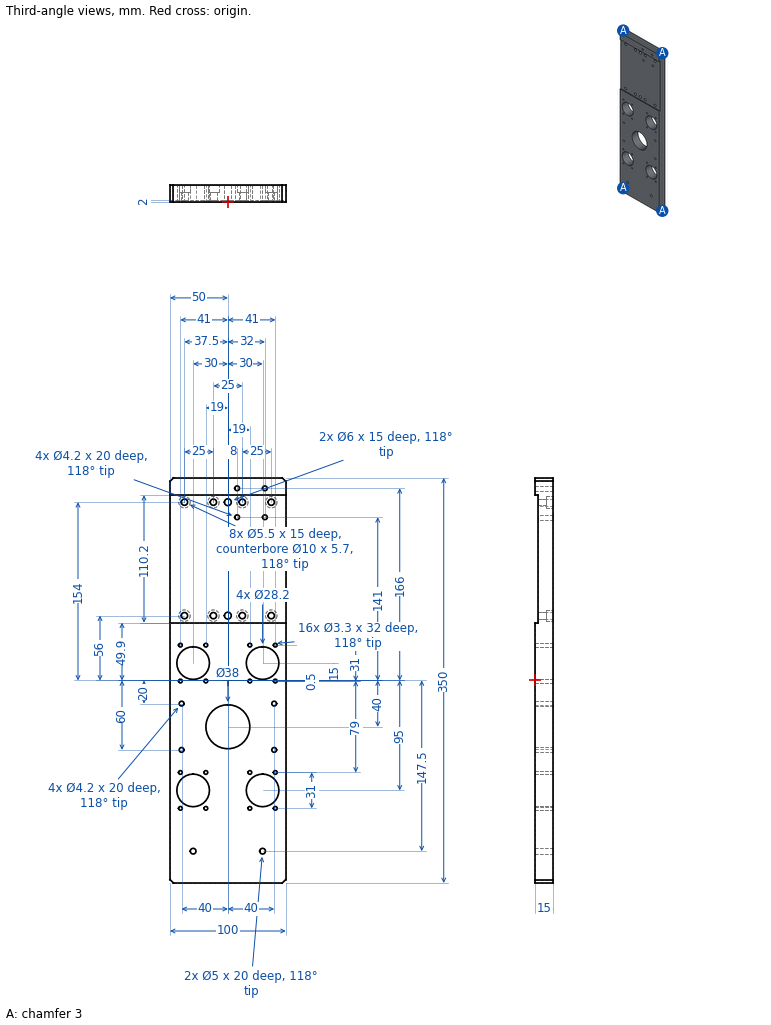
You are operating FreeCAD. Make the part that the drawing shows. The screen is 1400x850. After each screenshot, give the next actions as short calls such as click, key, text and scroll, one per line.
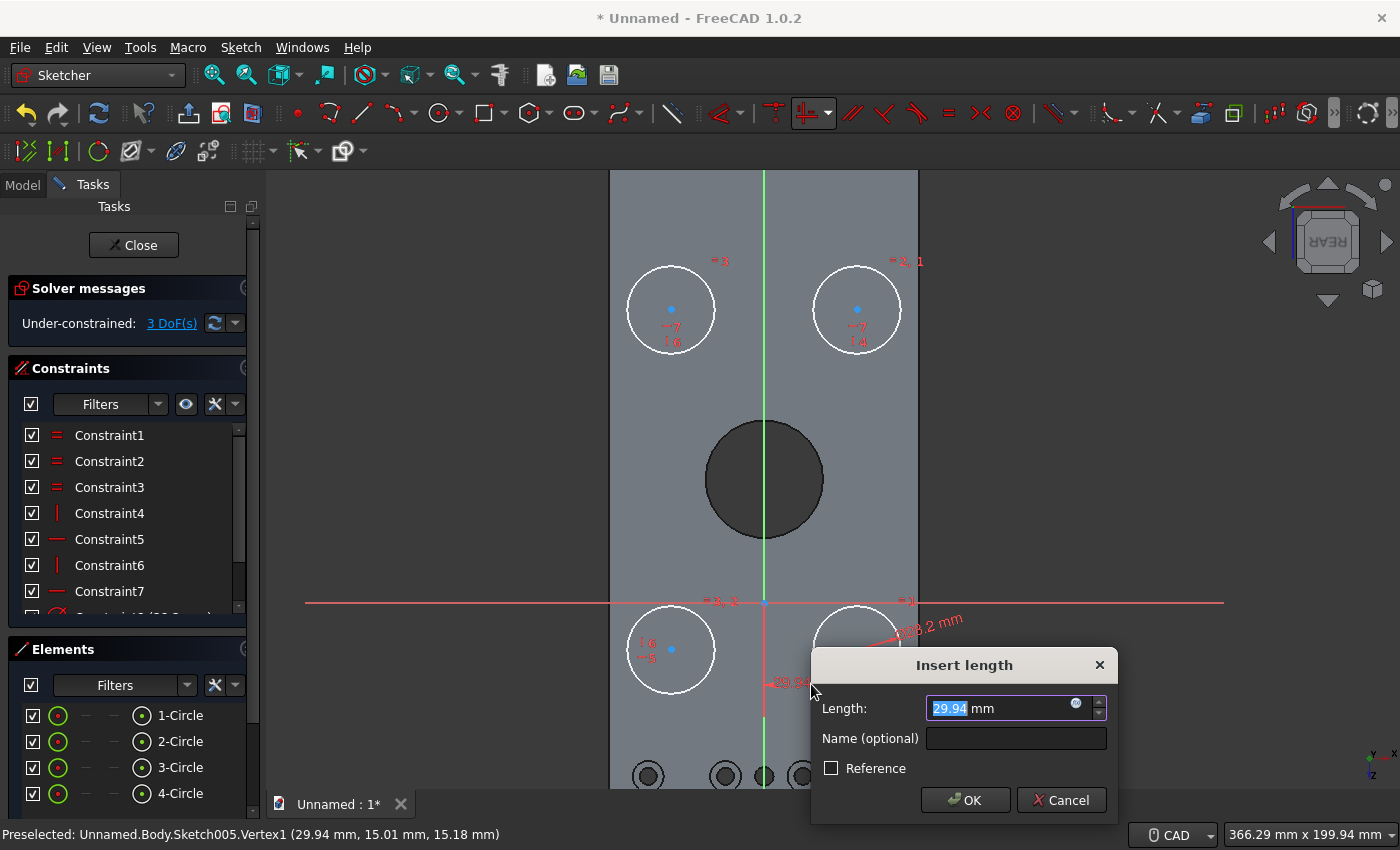
text(30)
key(Return)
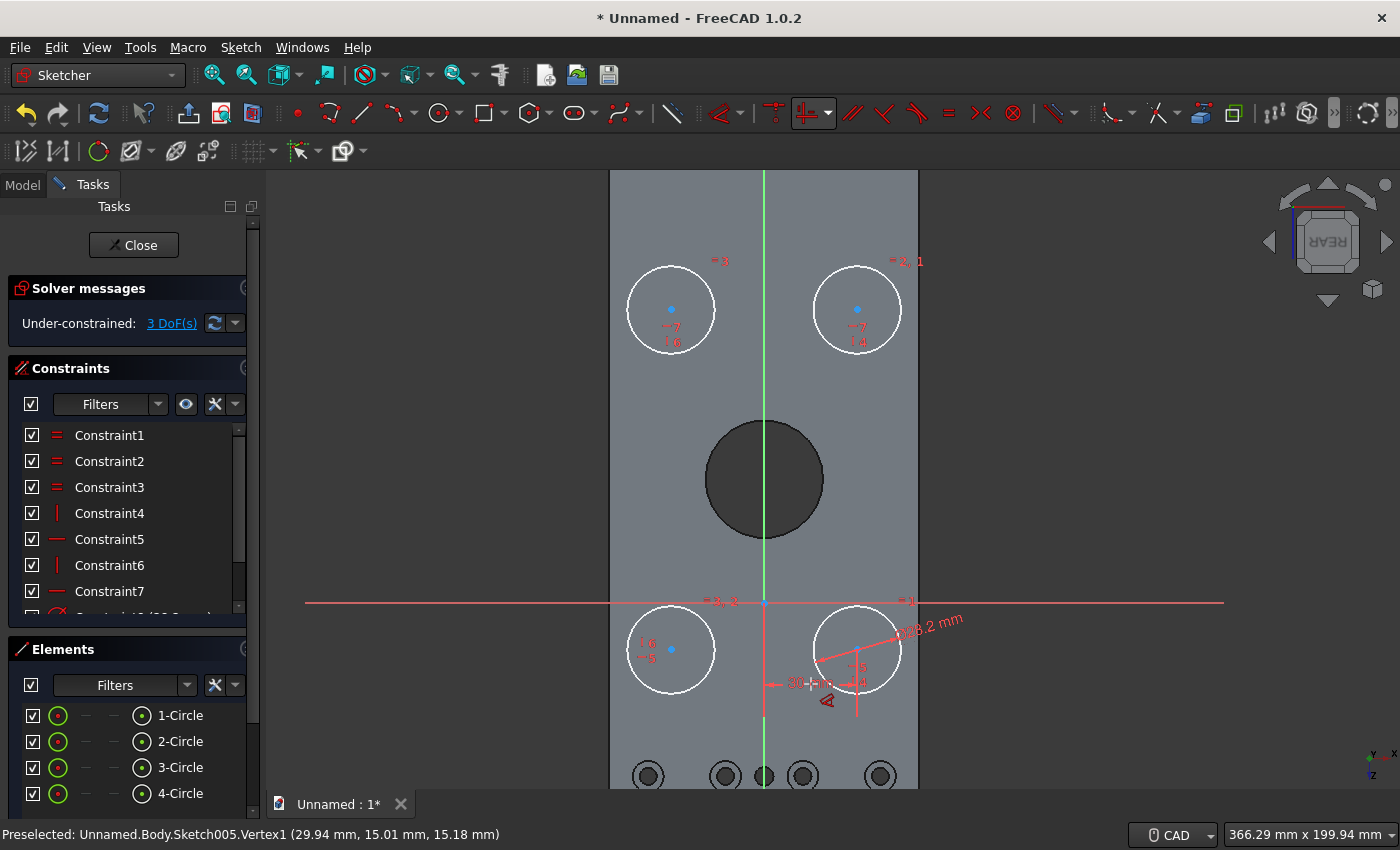
click(857, 650)
click(730, 627)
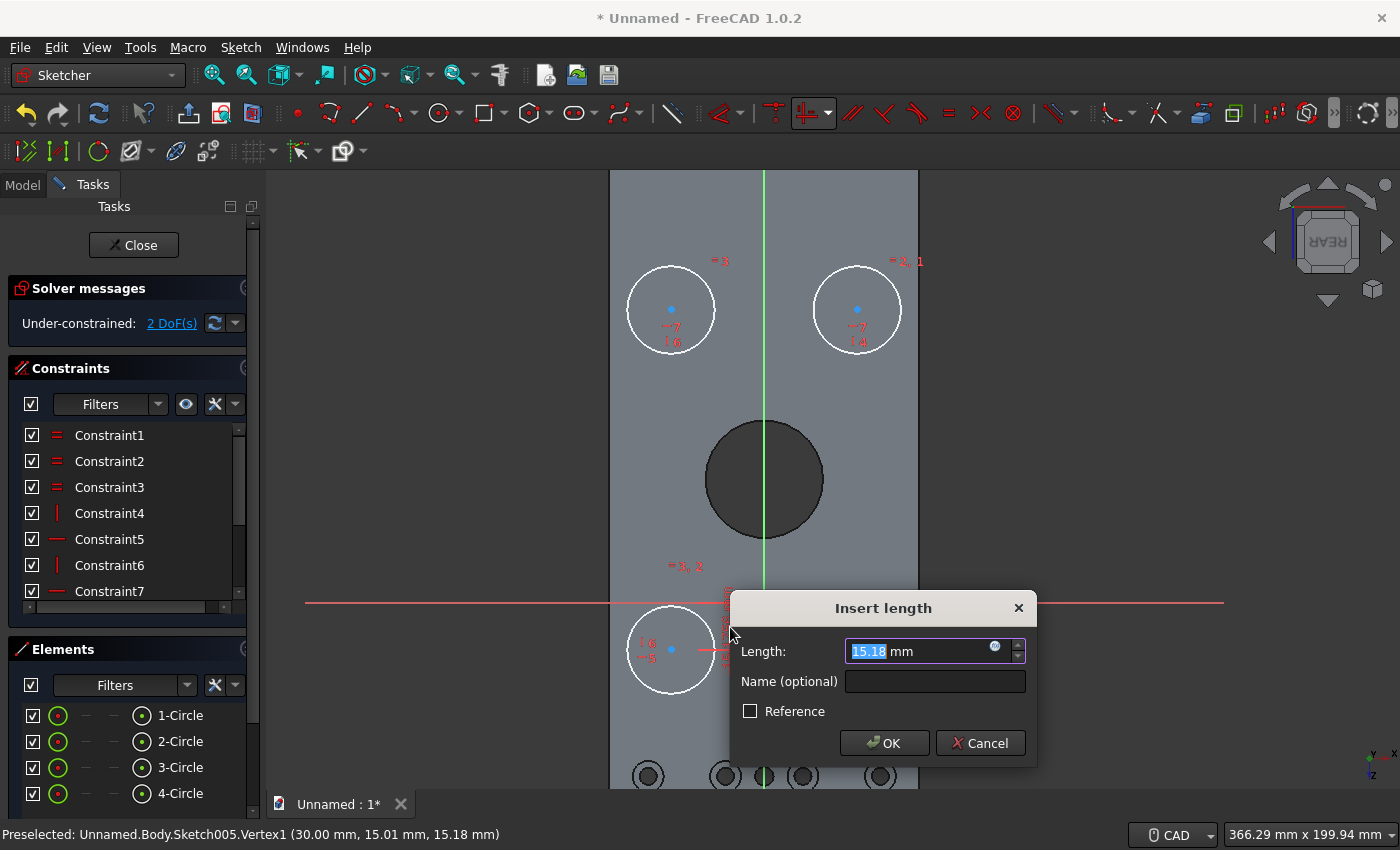
text(15)
key(Return)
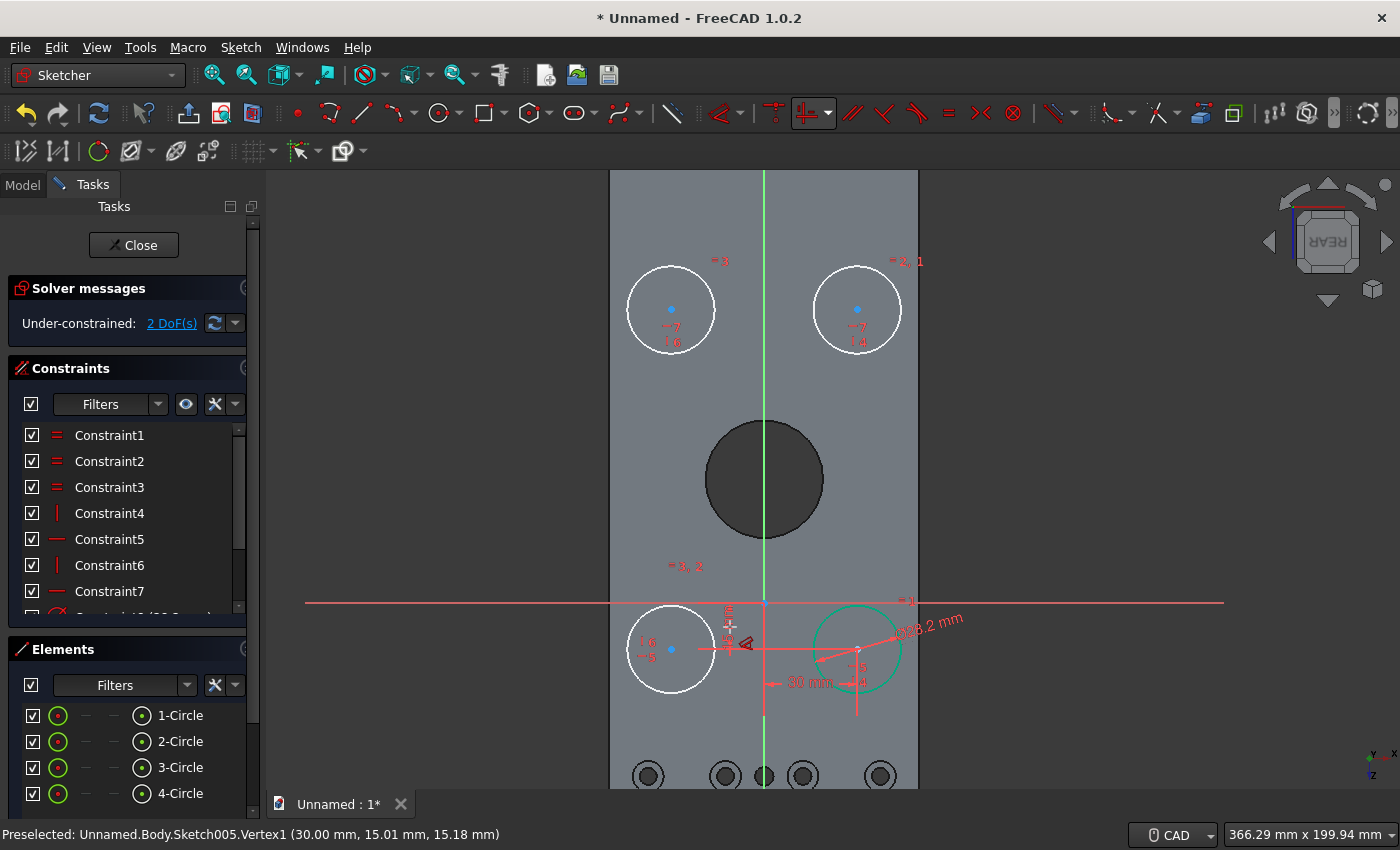
click(857, 310)
click(891, 457)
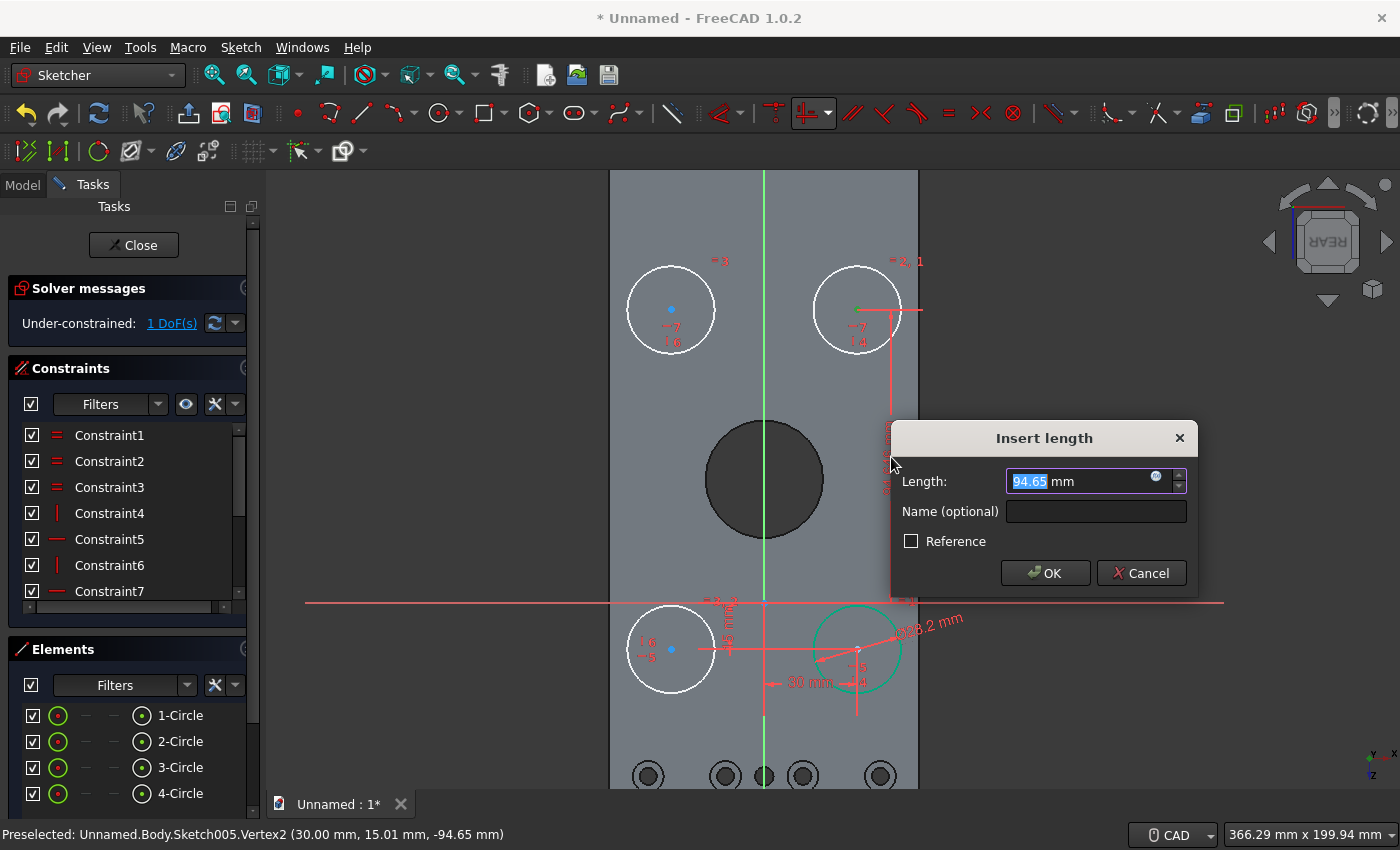
text(95)
key(Return)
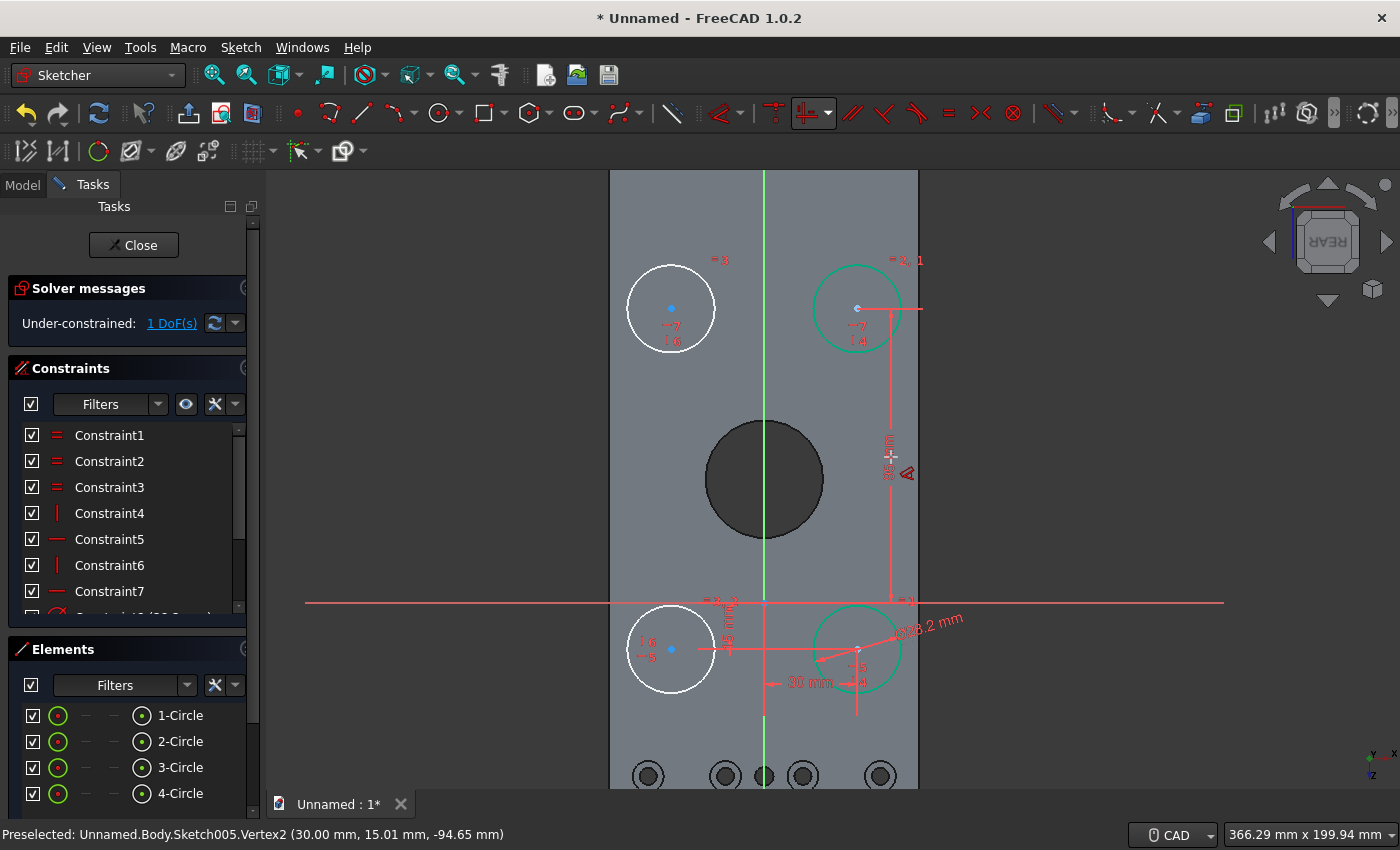
click(671, 649)
click(718, 683)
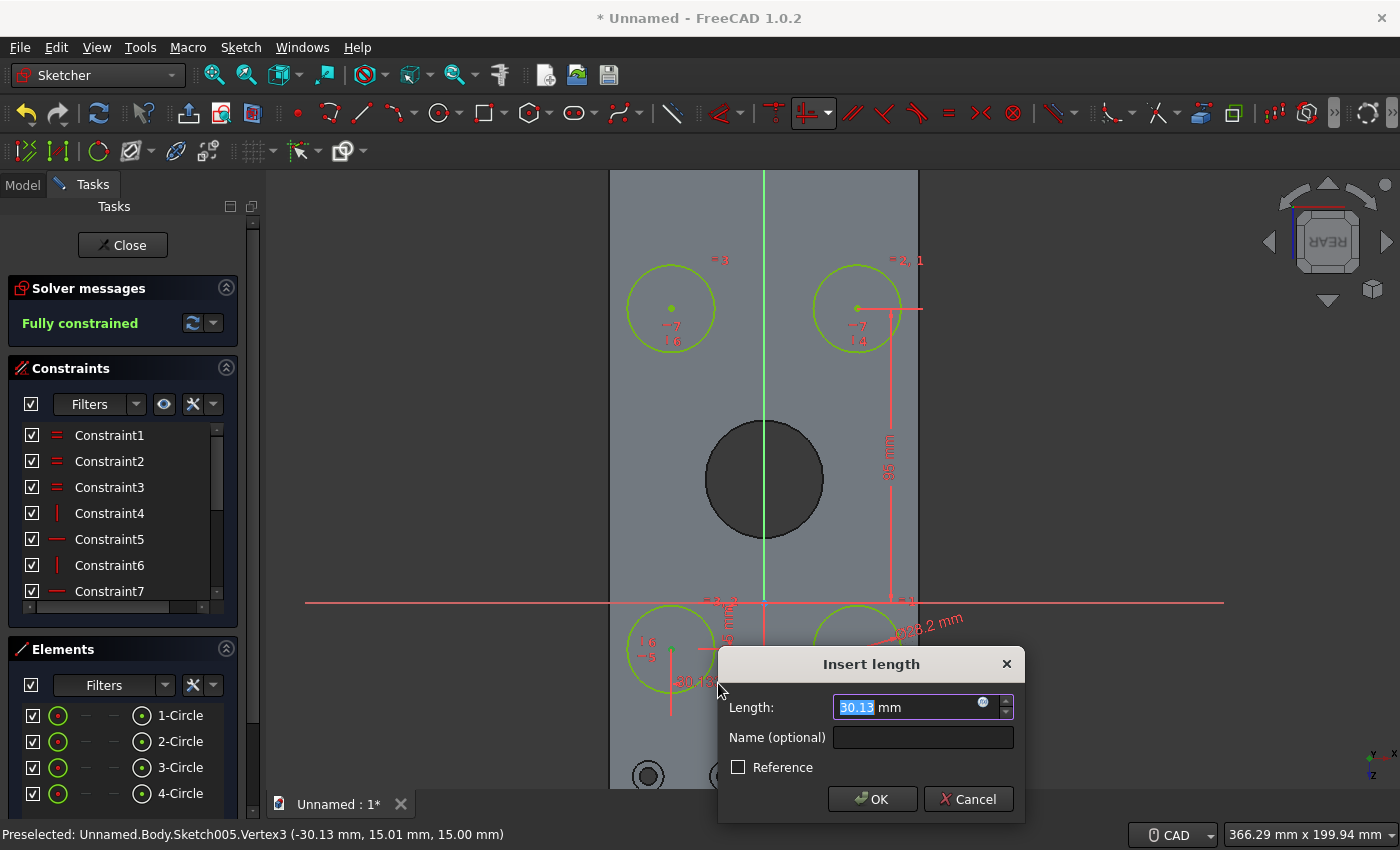
text(30)
key(Return)
key(Escape)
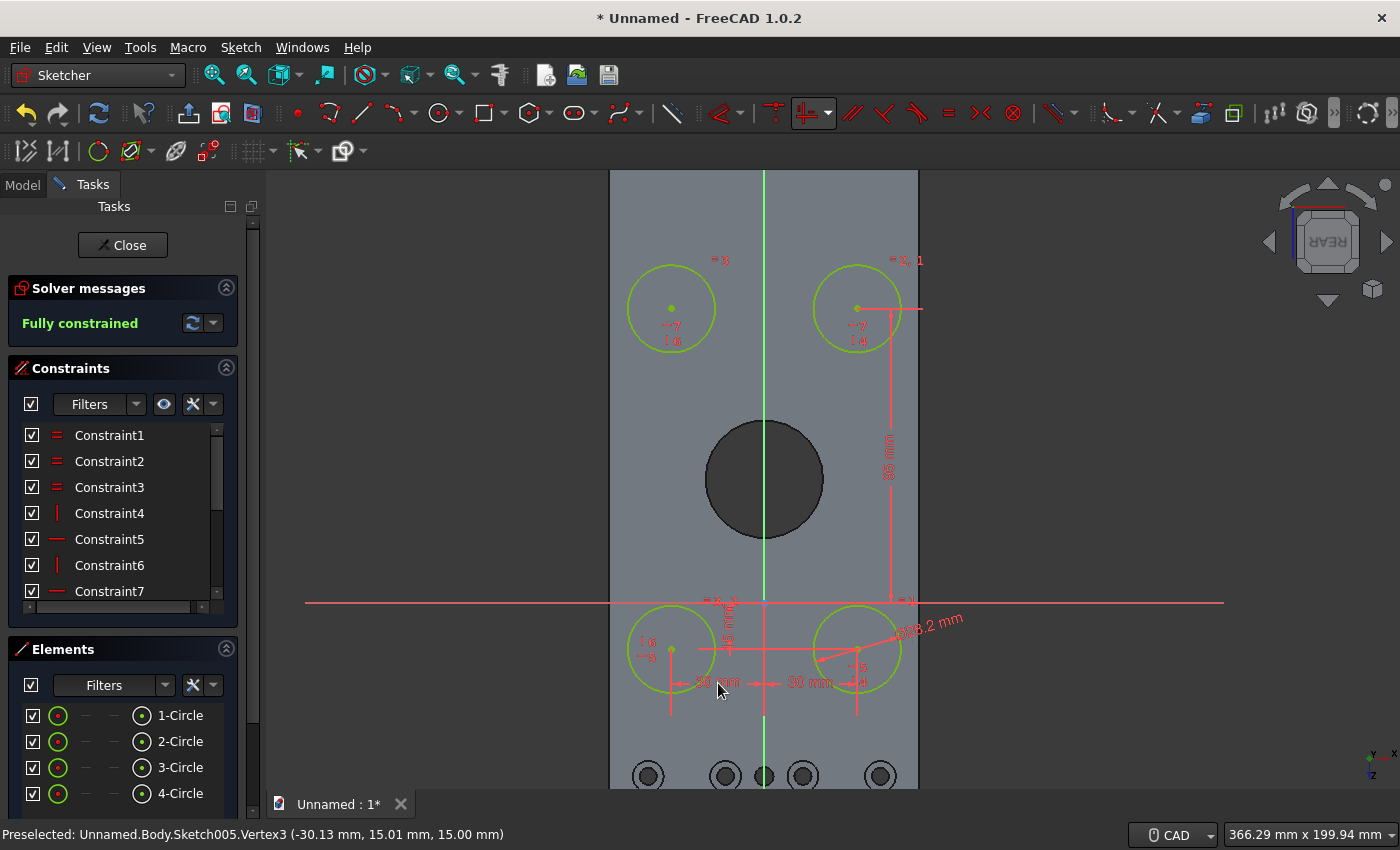
click(123, 245)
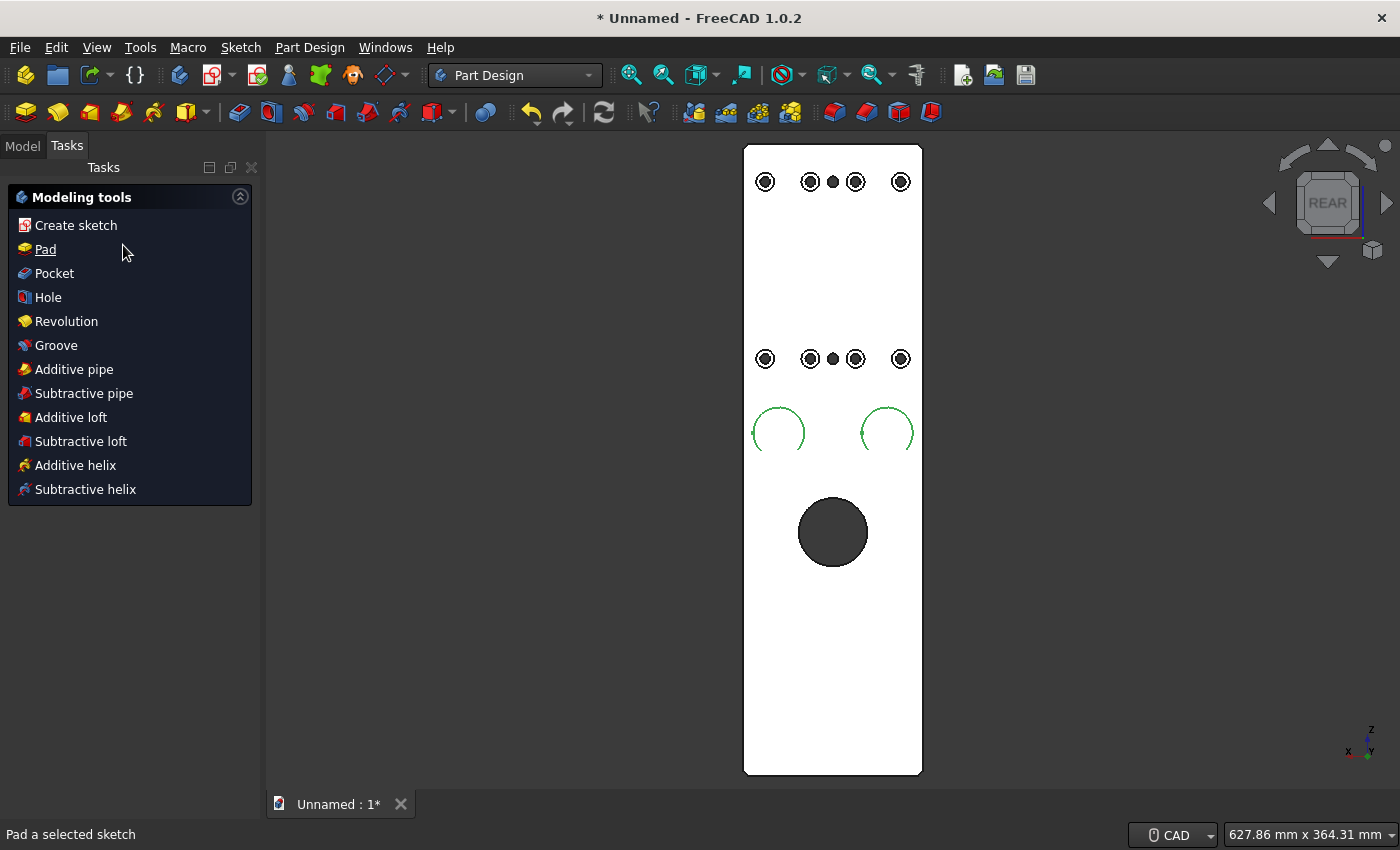
click(240, 112)